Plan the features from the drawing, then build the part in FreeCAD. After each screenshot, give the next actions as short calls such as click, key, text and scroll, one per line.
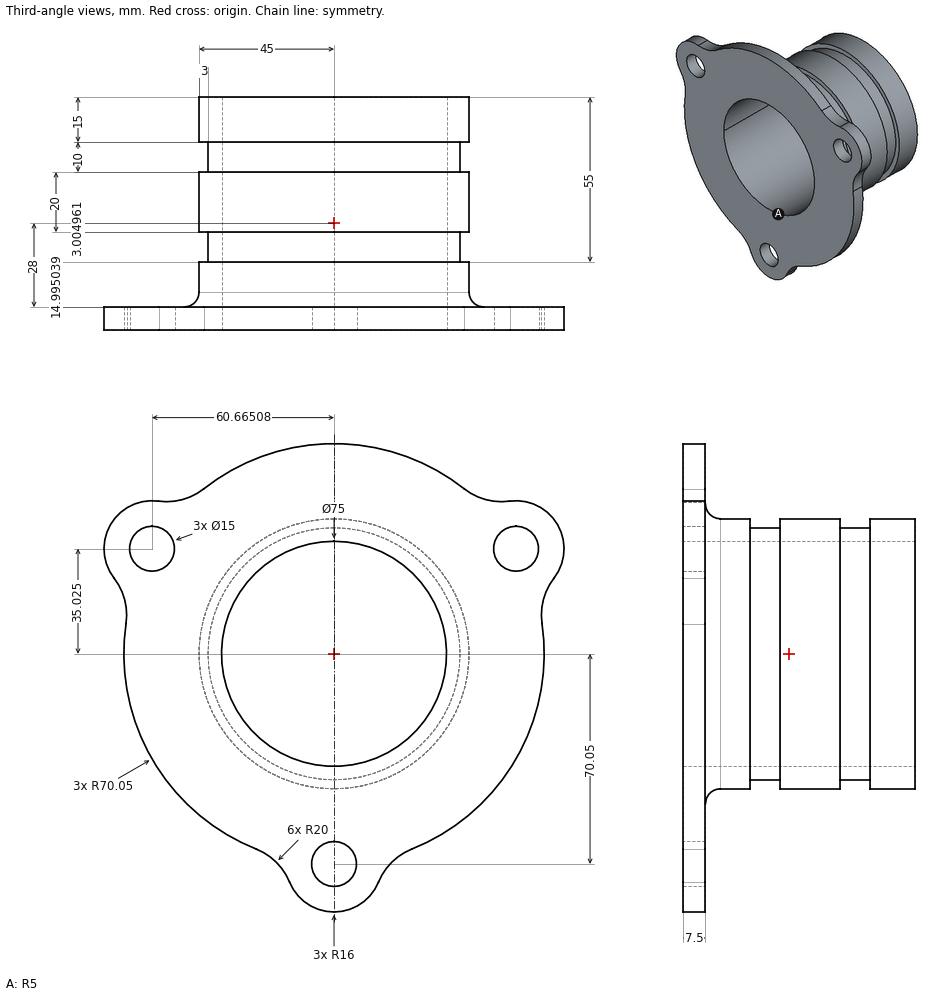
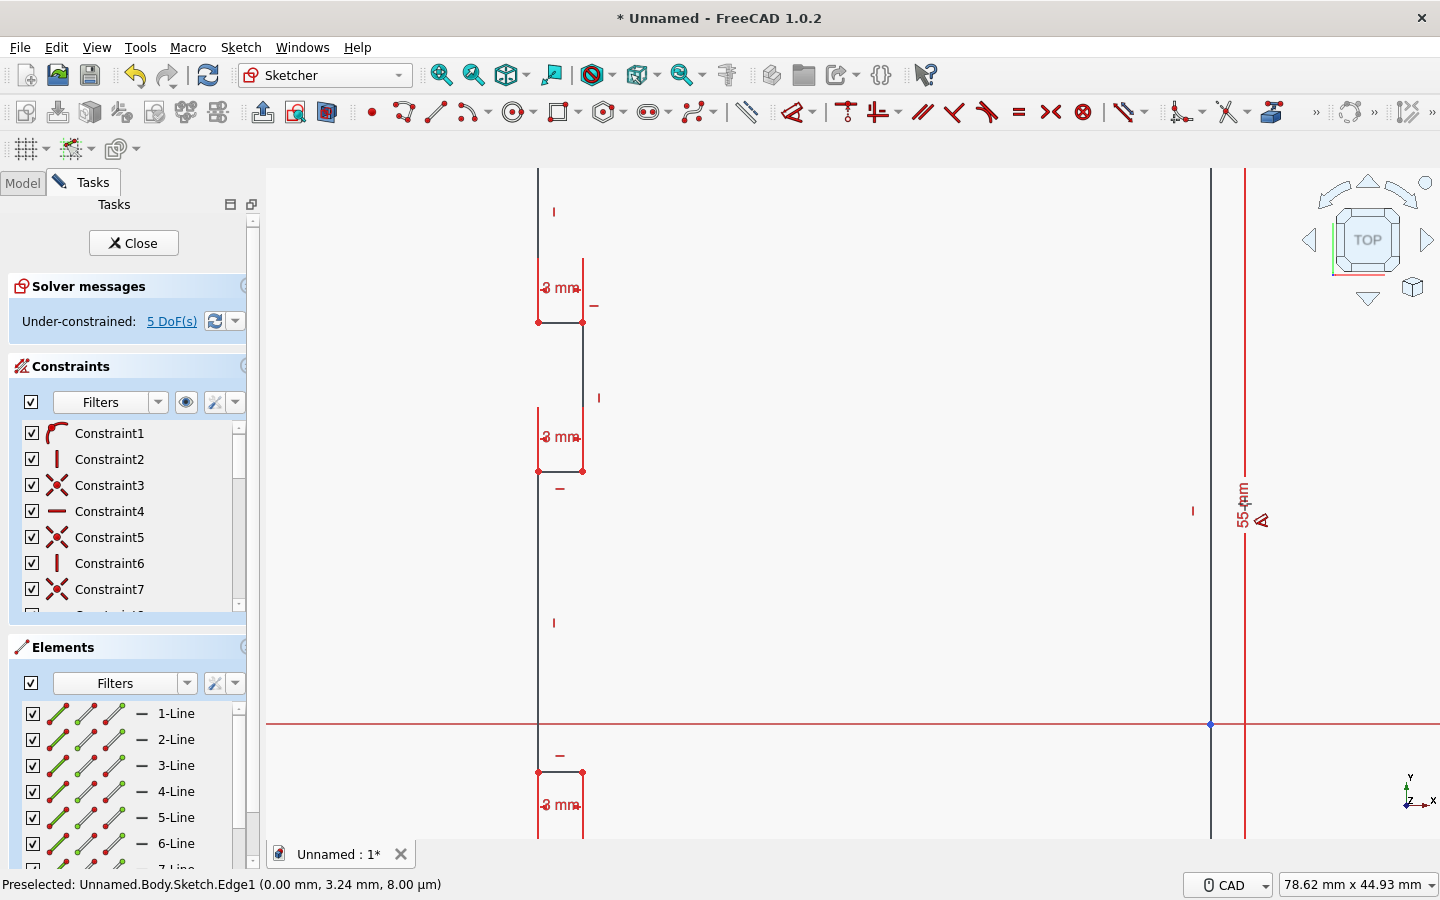
scroll(675, 498, down, 3)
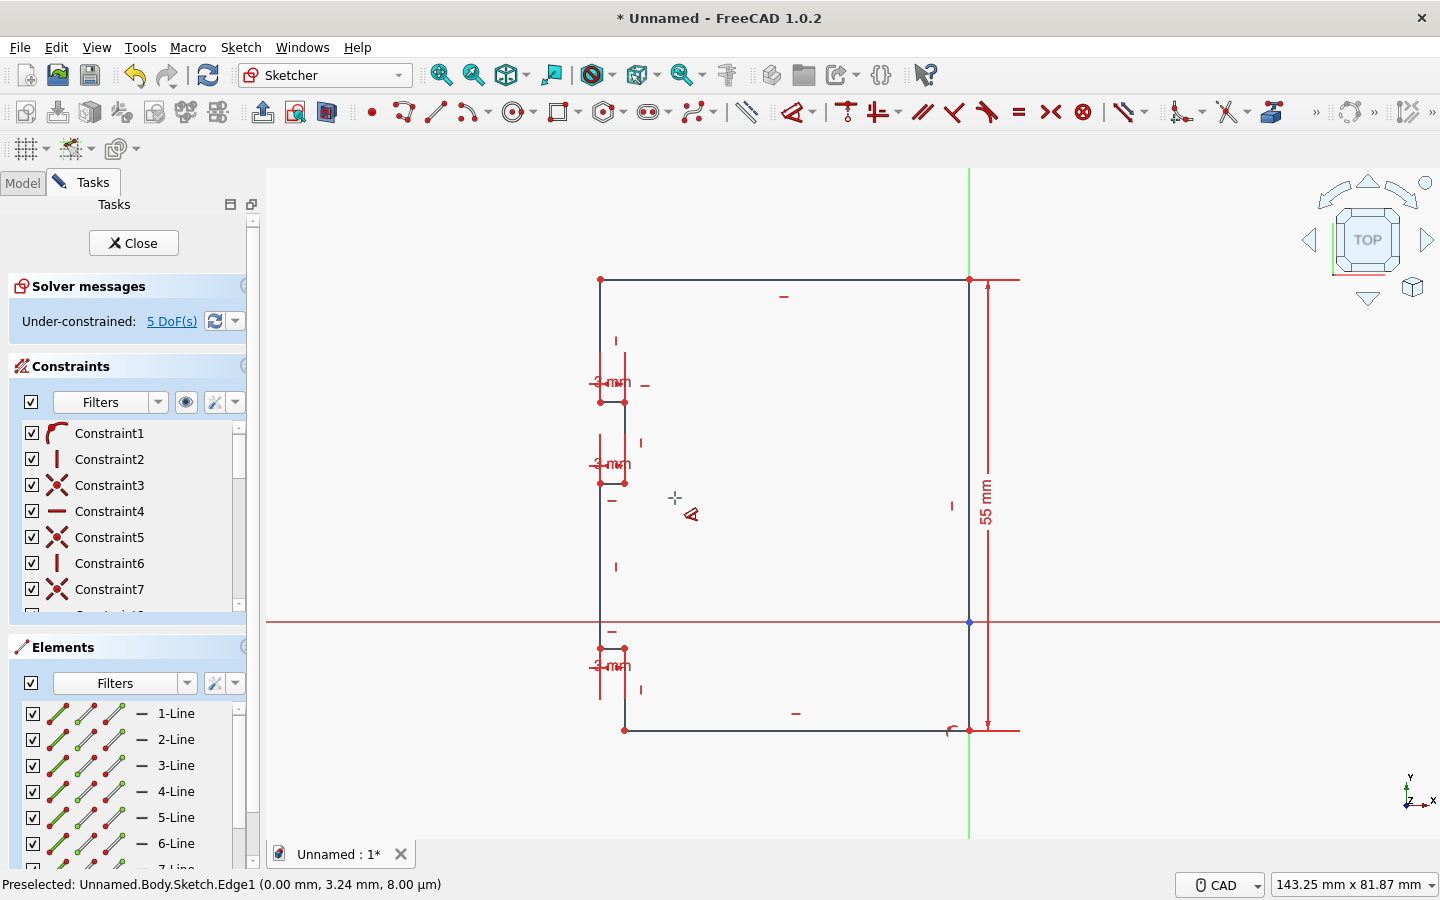
click(858, 280)
click(785, 246)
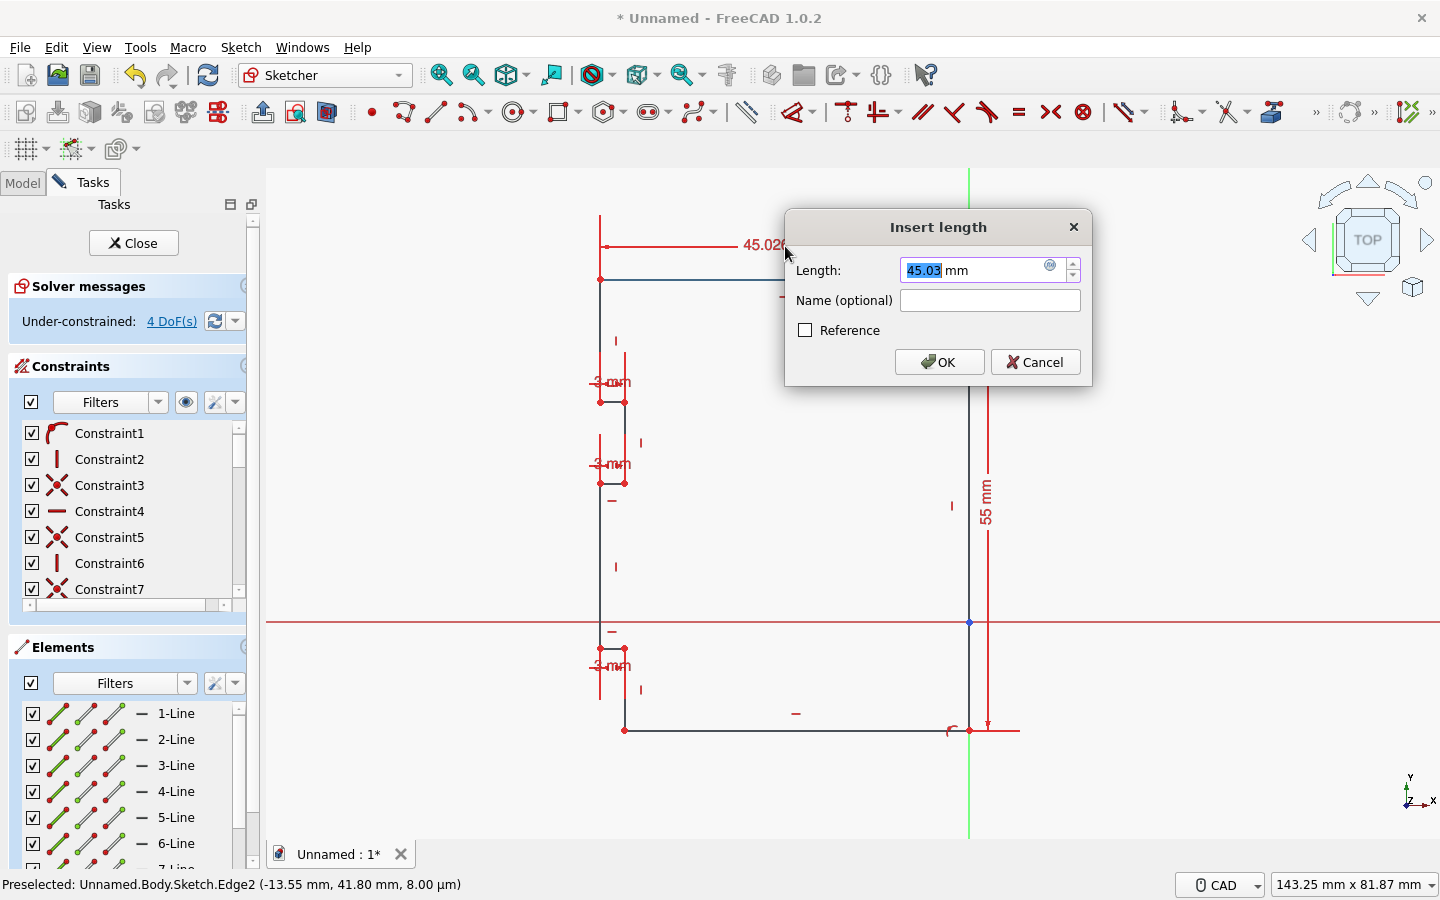
text(45)
key(Return)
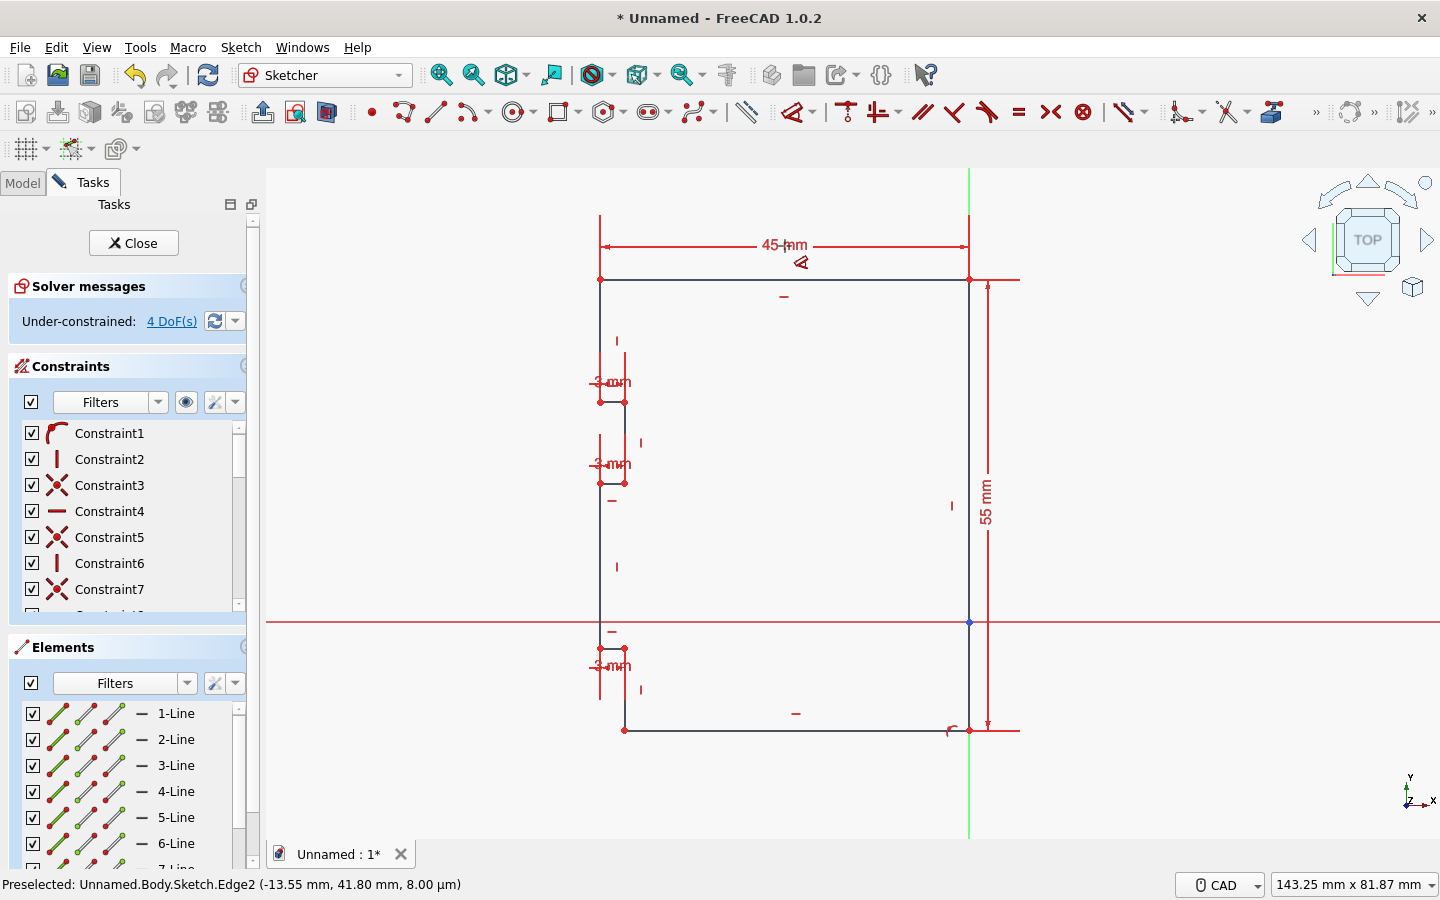
click(600, 317)
click(566, 341)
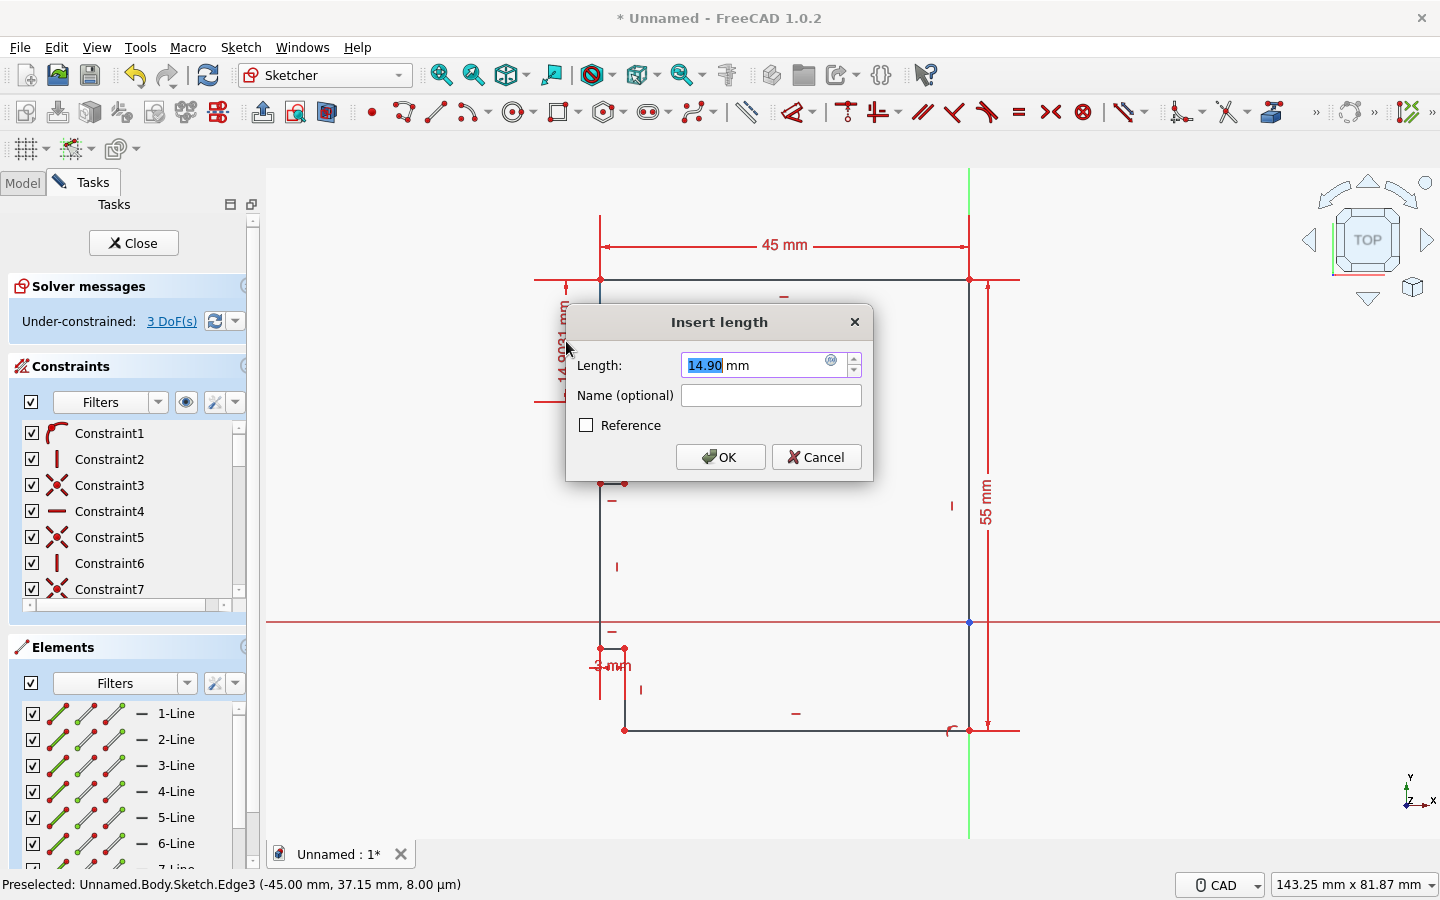
text(15)
key(Return)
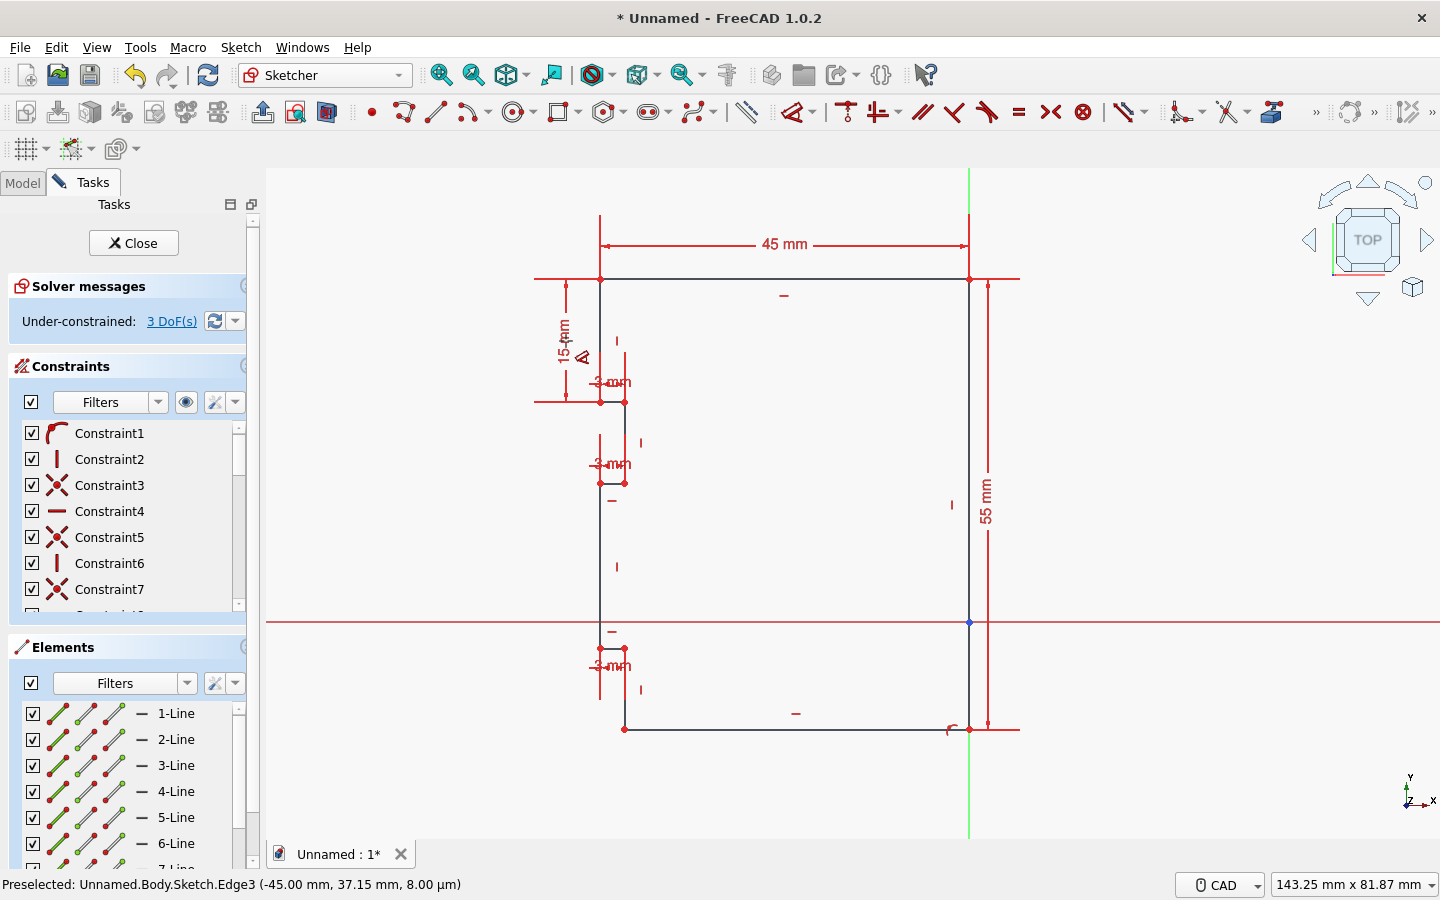
click(625, 427)
click(591, 443)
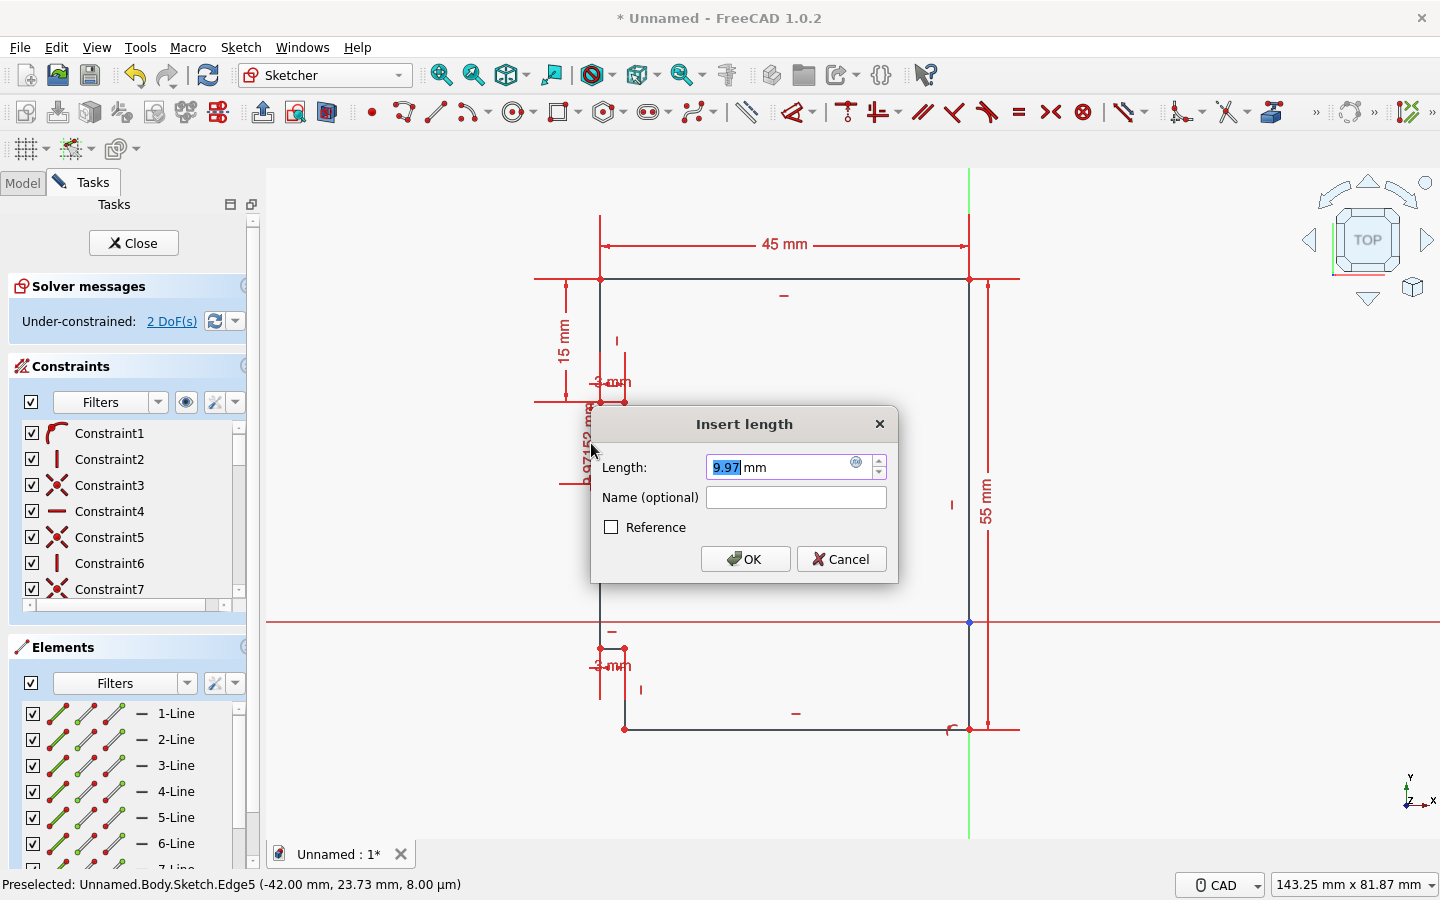
text(10)
key(Return)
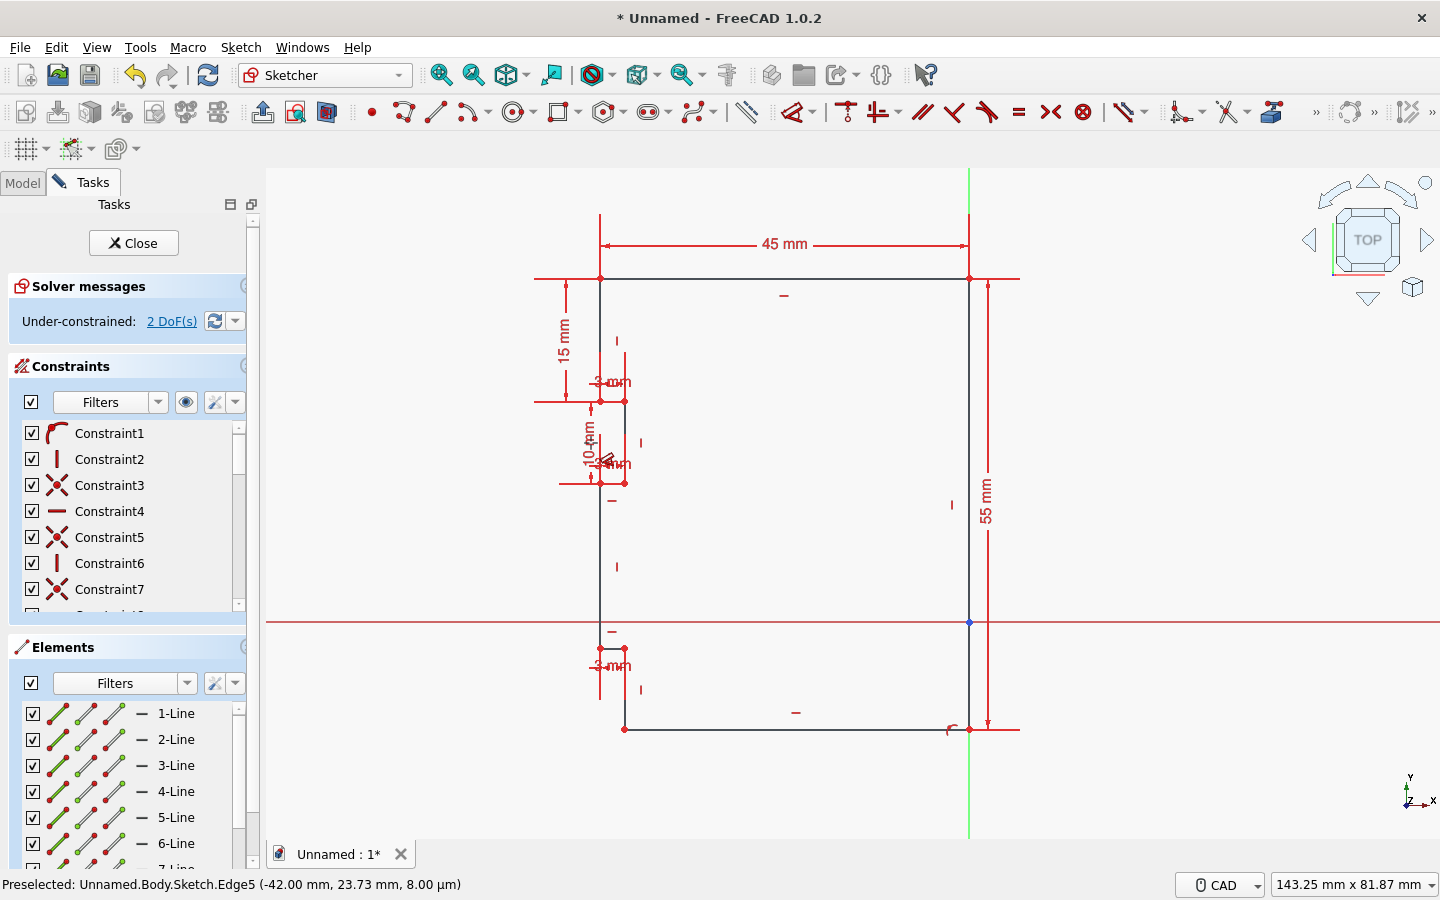
click(600, 533)
click(566, 566)